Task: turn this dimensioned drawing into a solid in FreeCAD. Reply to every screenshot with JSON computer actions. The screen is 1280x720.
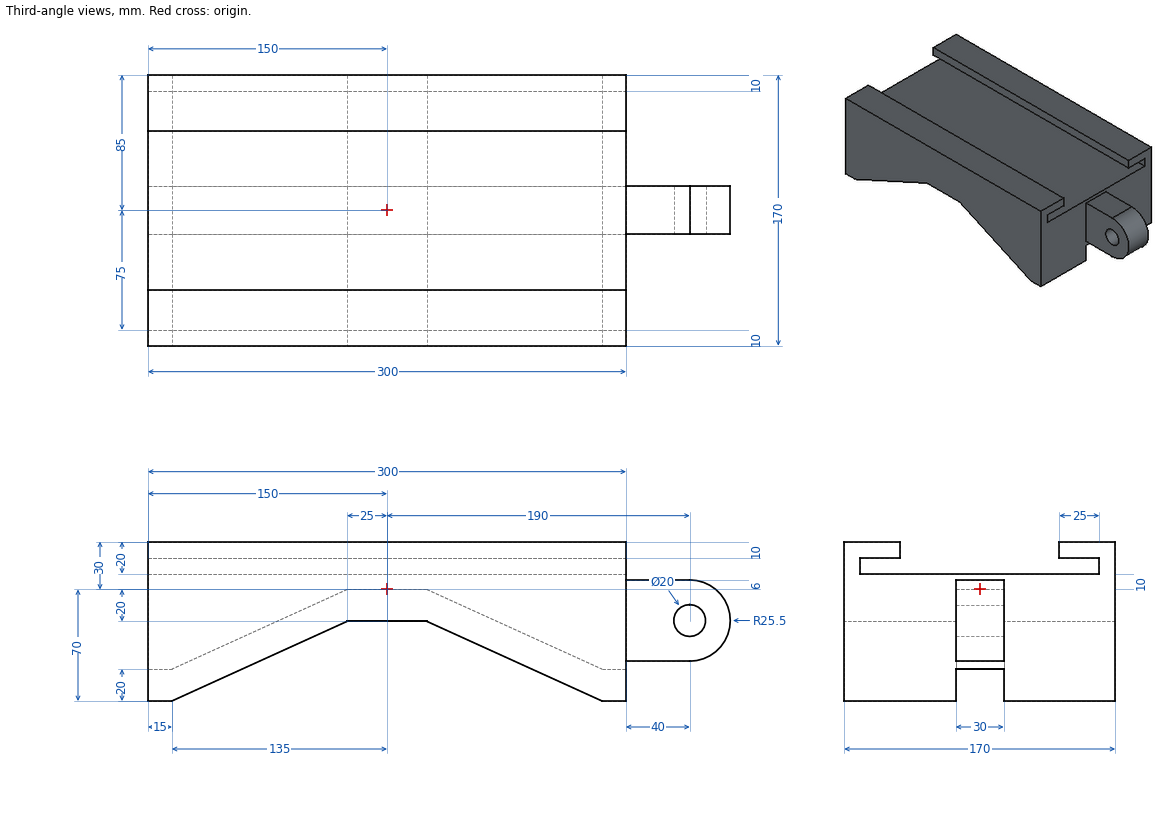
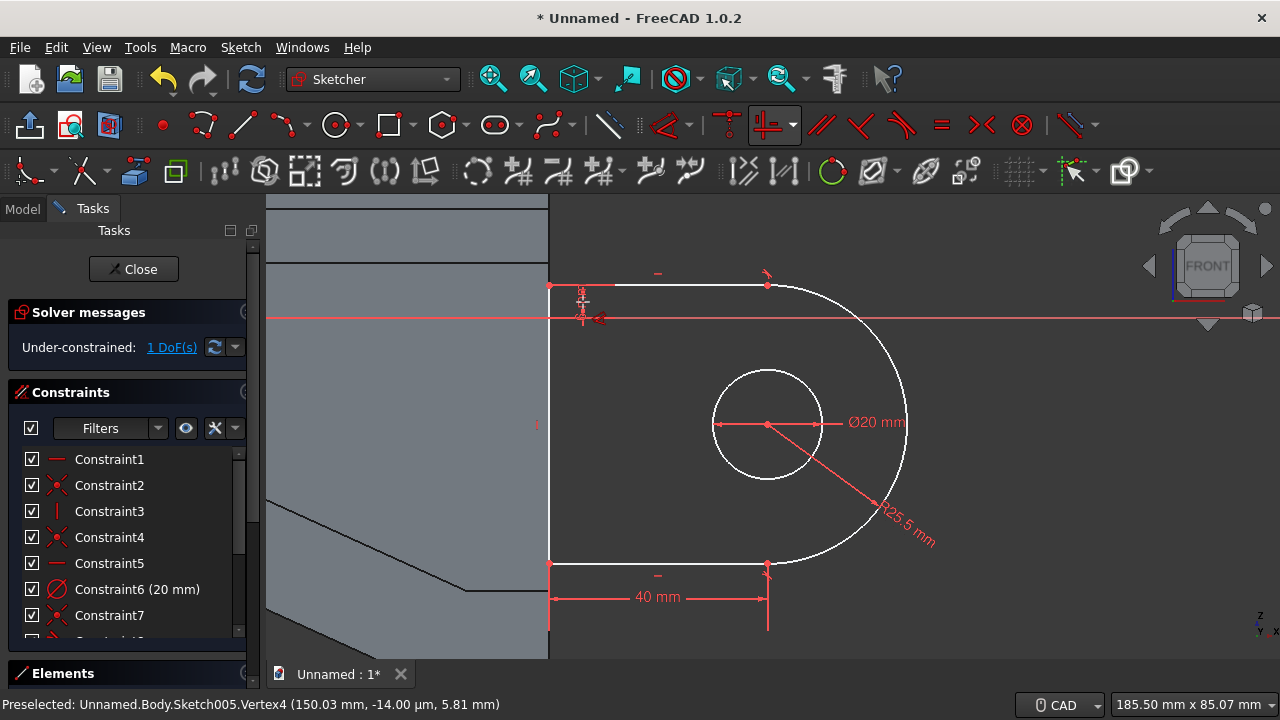
{"action": "left_click", "coordinate": [768, 424]}
{"action": "left_click", "coordinate": [422, 284]}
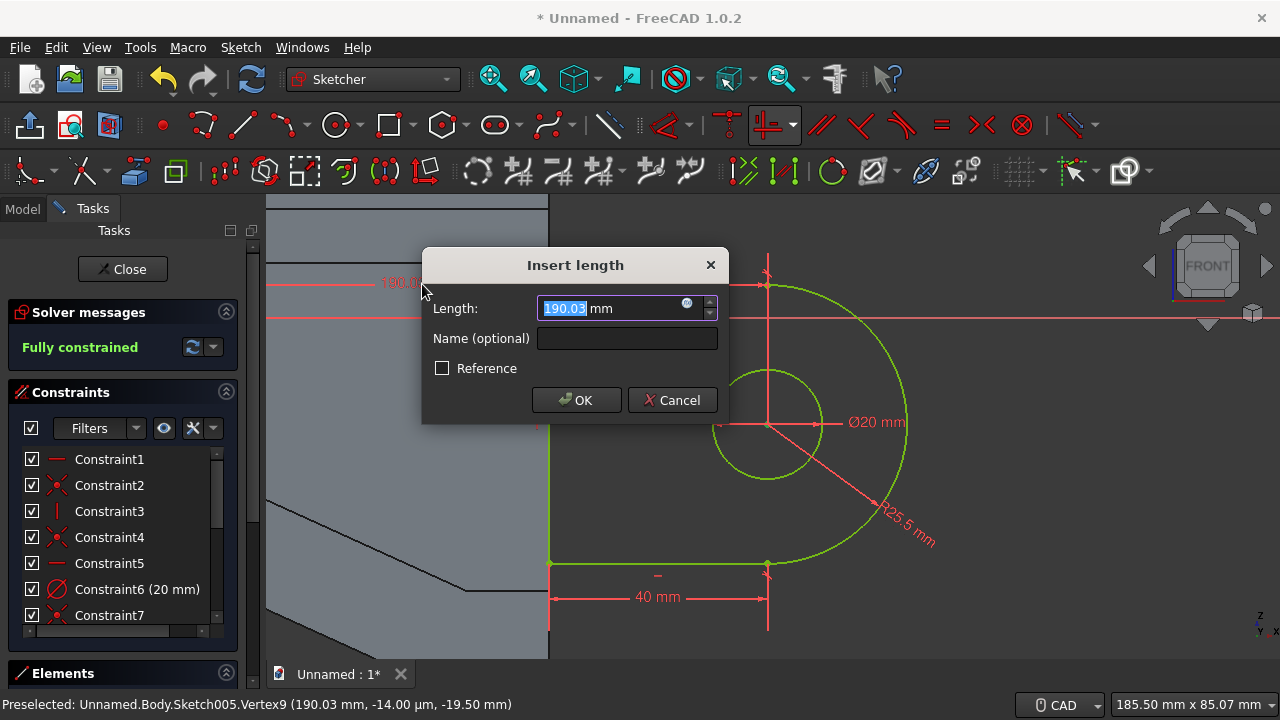
{"action": "type", "text": "190"}
{"action": "key", "text": "Return"}
{"action": "key", "text": "Escape"}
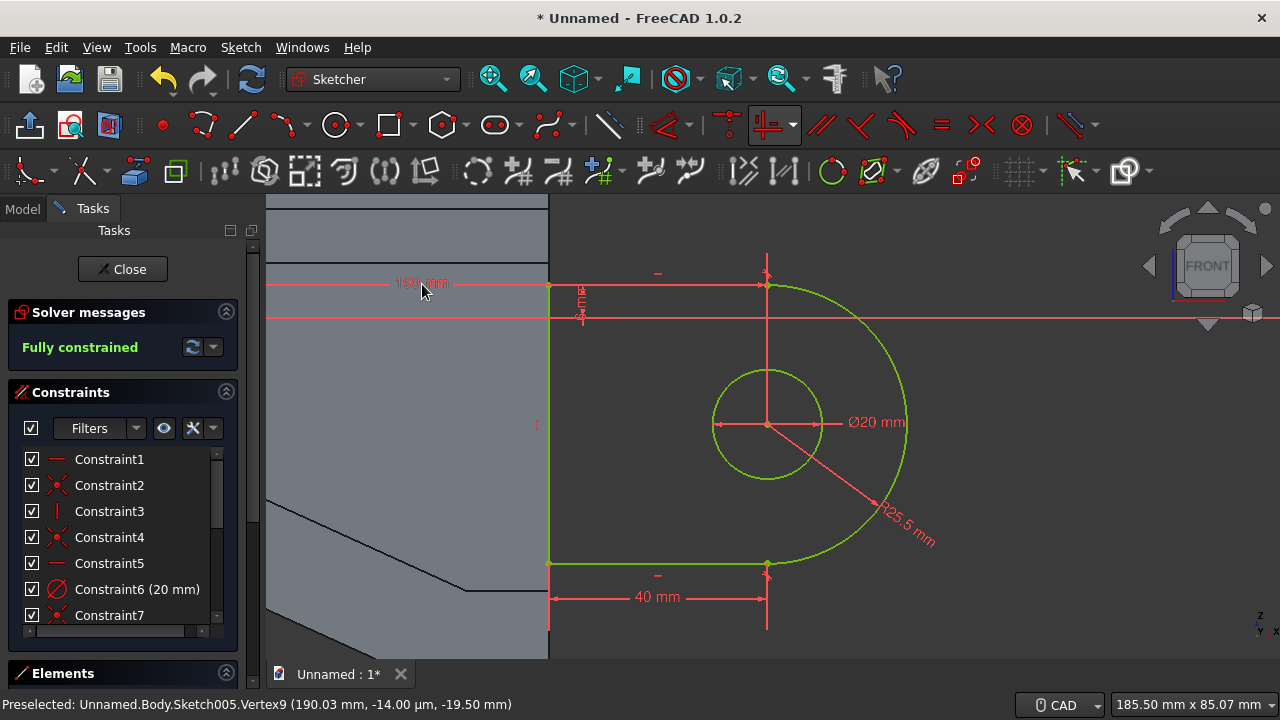
{"action": "left_click", "coordinate": [123, 269]}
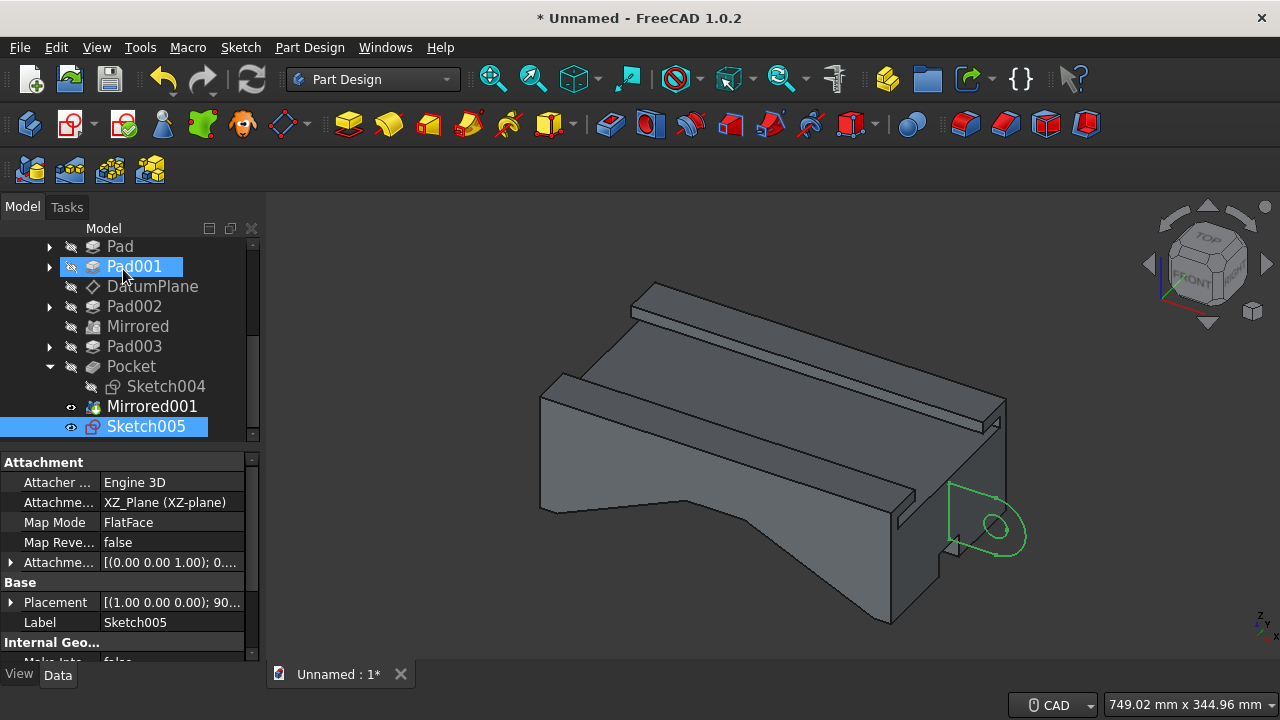
{"action": "left_click", "coordinate": [350, 124]}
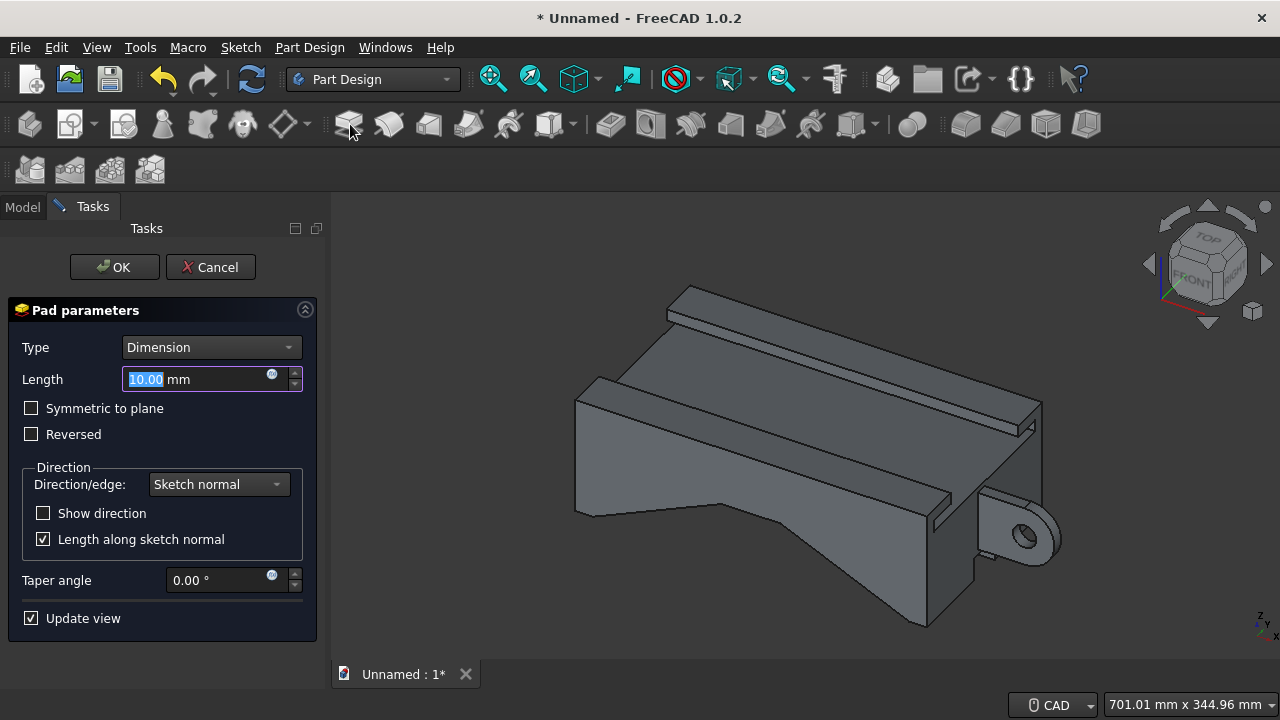
{"action": "type", "text": "30"}
{"action": "key", "text": "Tab"}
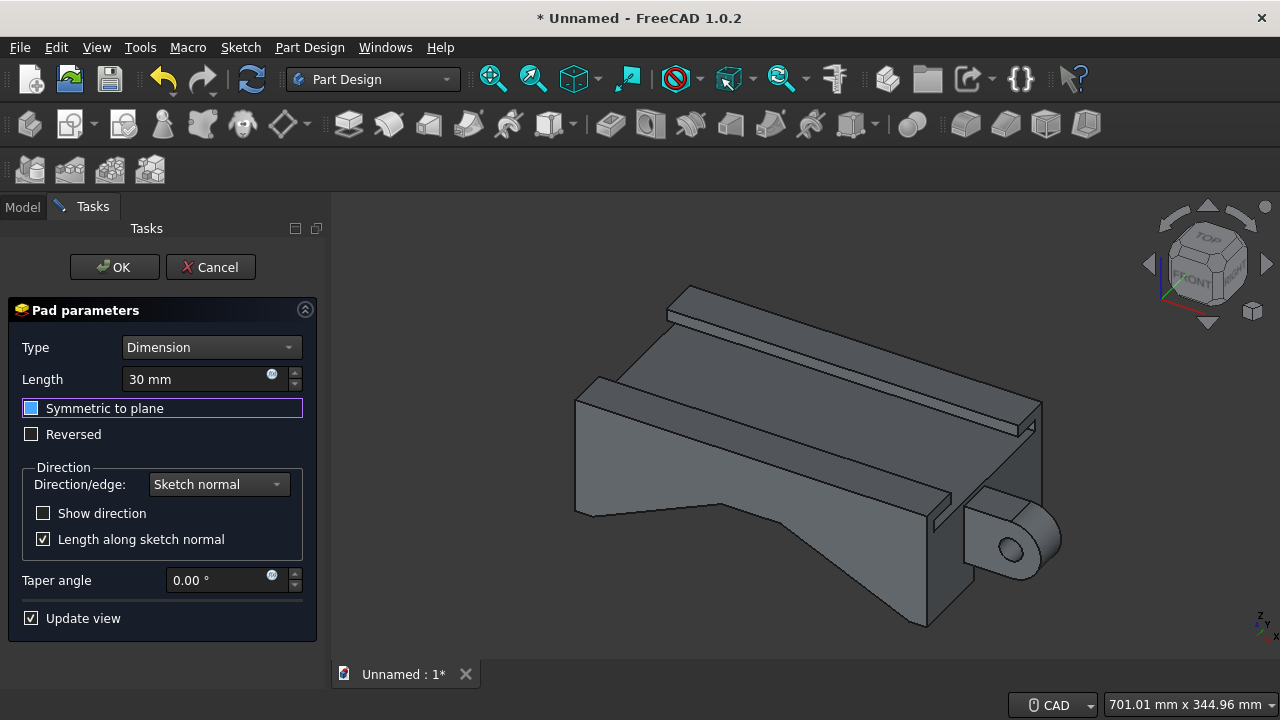
{"action": "left_click", "coordinate": [30, 408]}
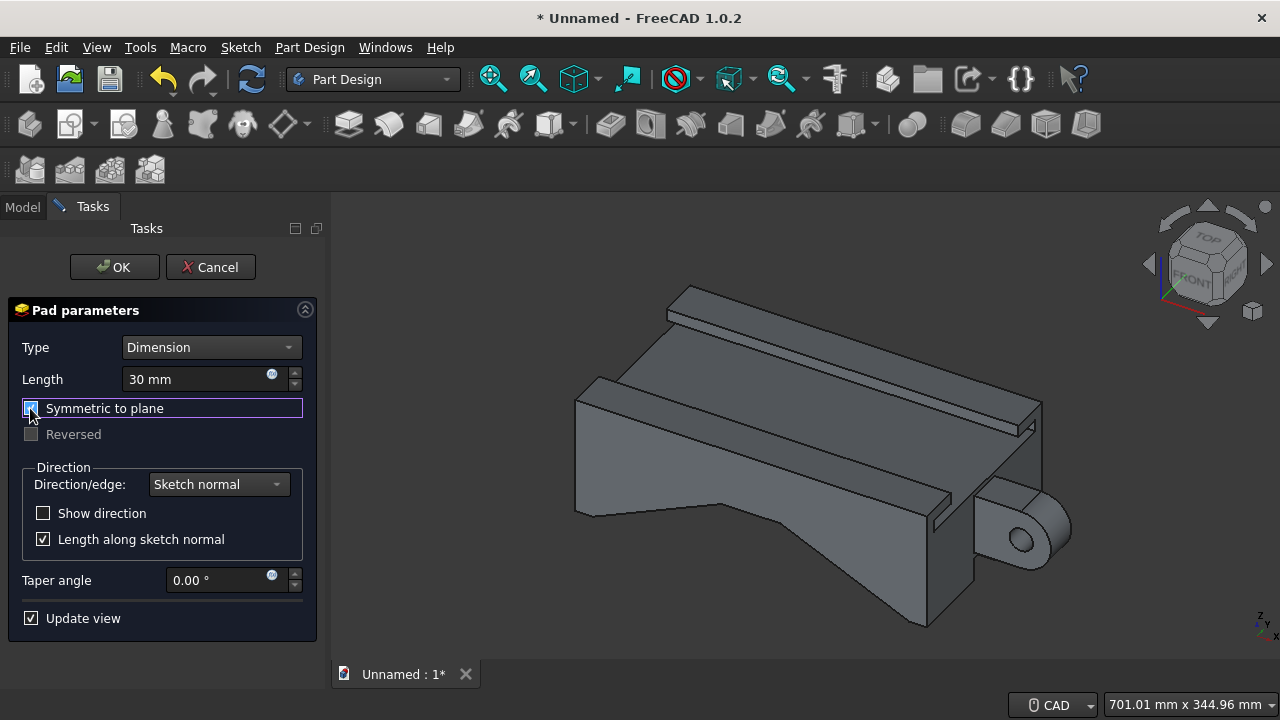
{"action": "left_click", "coordinate": [115, 267]}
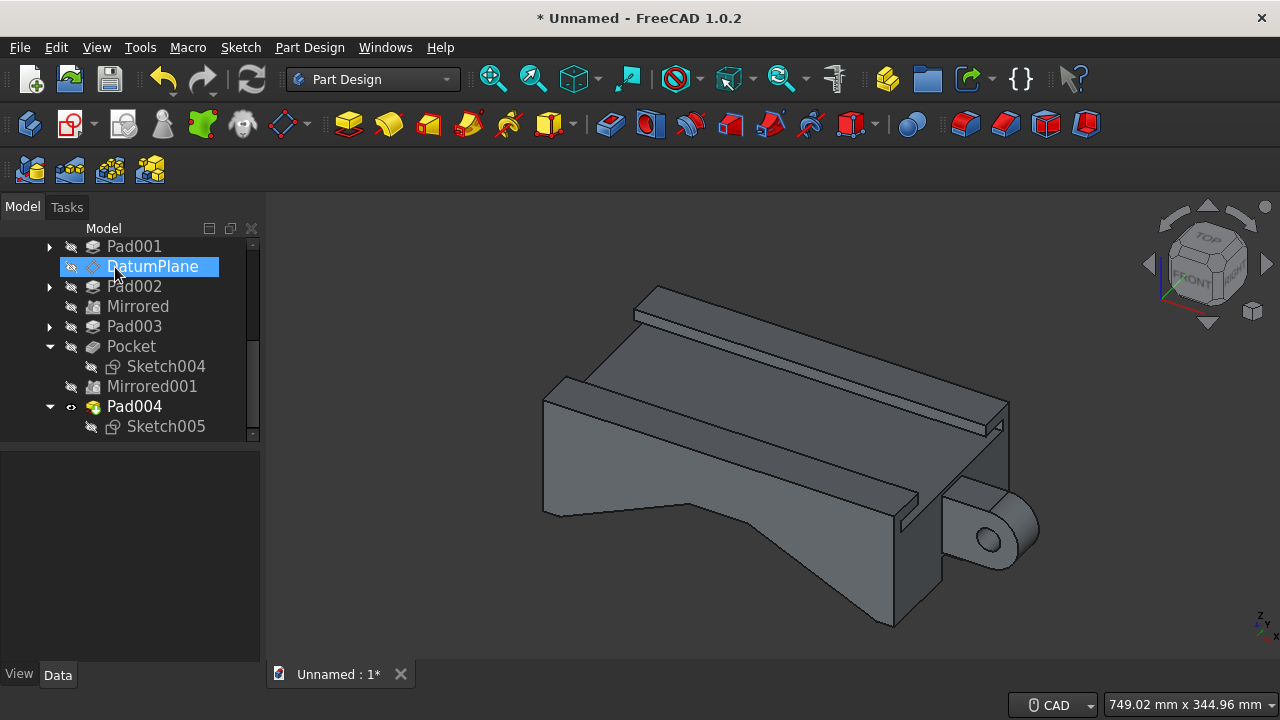
{"action": "key", "text": "0"}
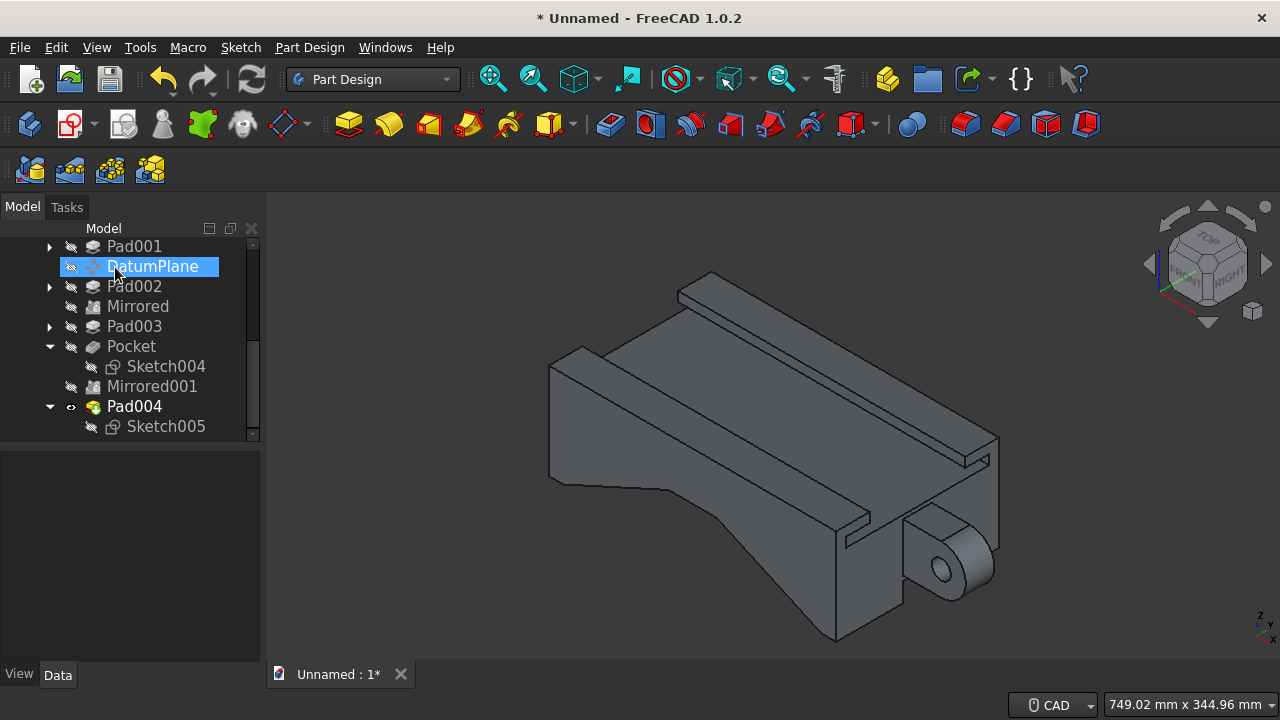
{"action": "key", "text": "v f"}